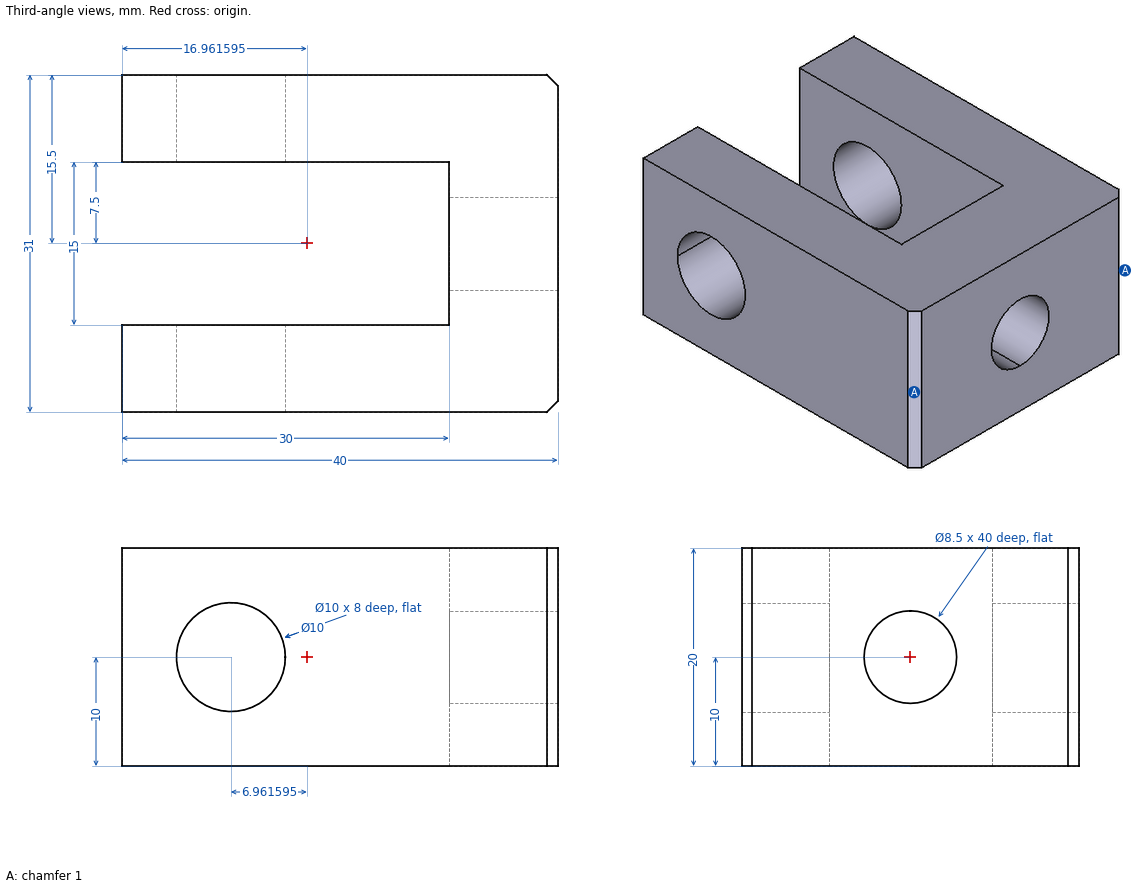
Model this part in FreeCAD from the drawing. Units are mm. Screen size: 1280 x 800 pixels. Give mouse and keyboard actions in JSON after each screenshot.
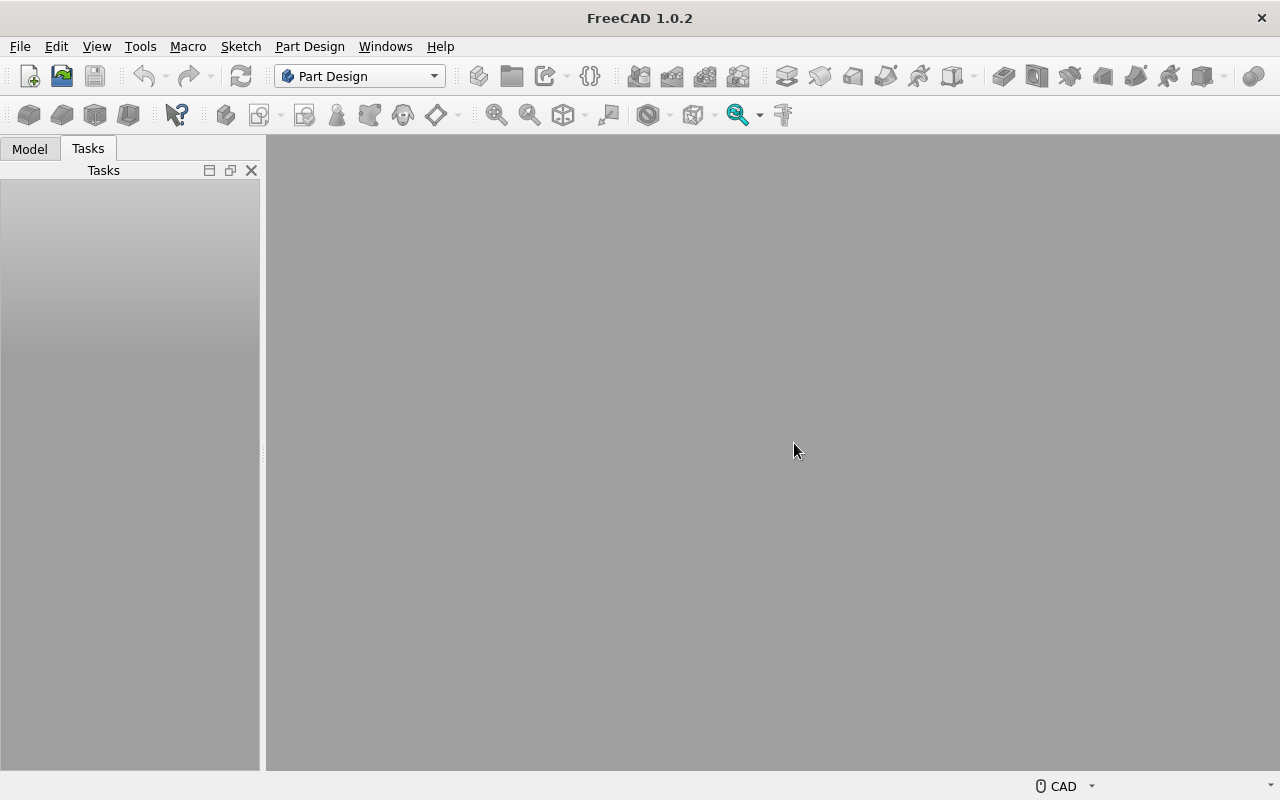
{"action": "left_click", "coordinate": [29, 76]}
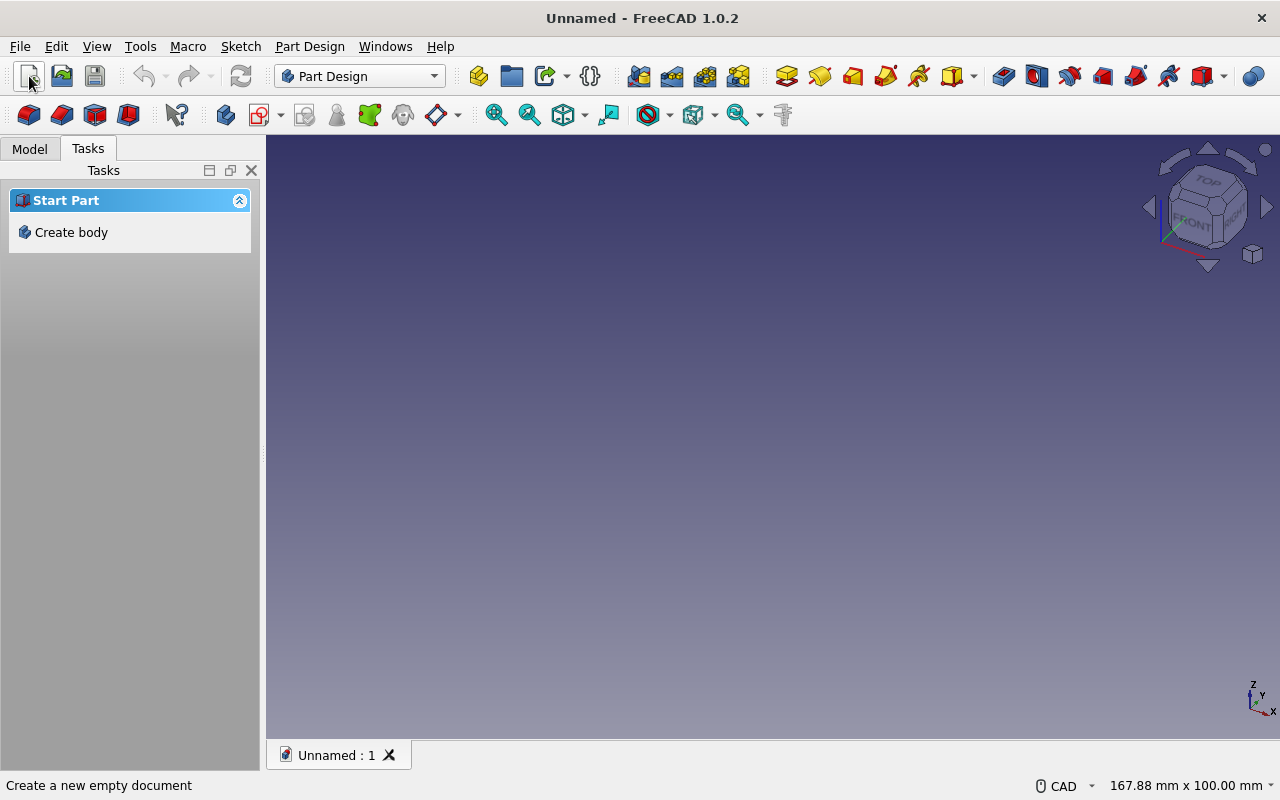
{"action": "left_click", "coordinate": [226, 116]}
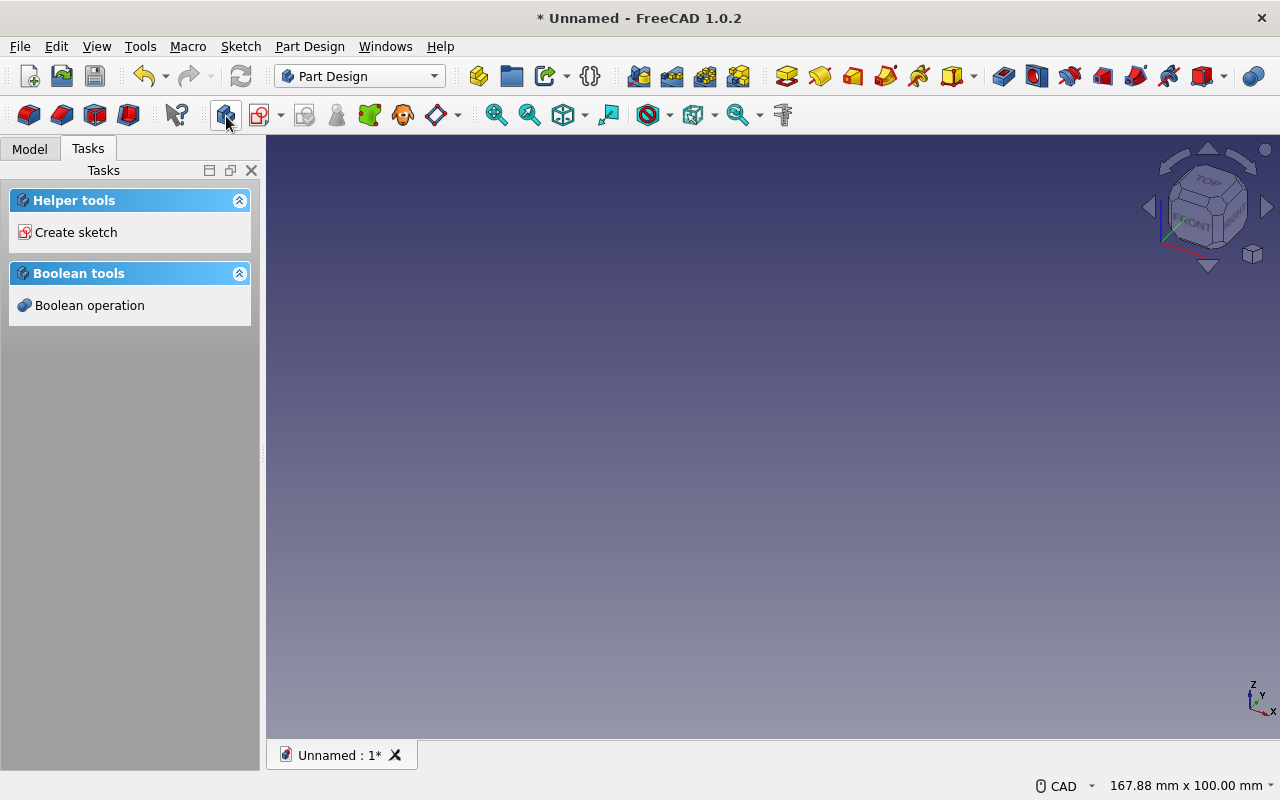
{"action": "left_click", "coordinate": [30, 148]}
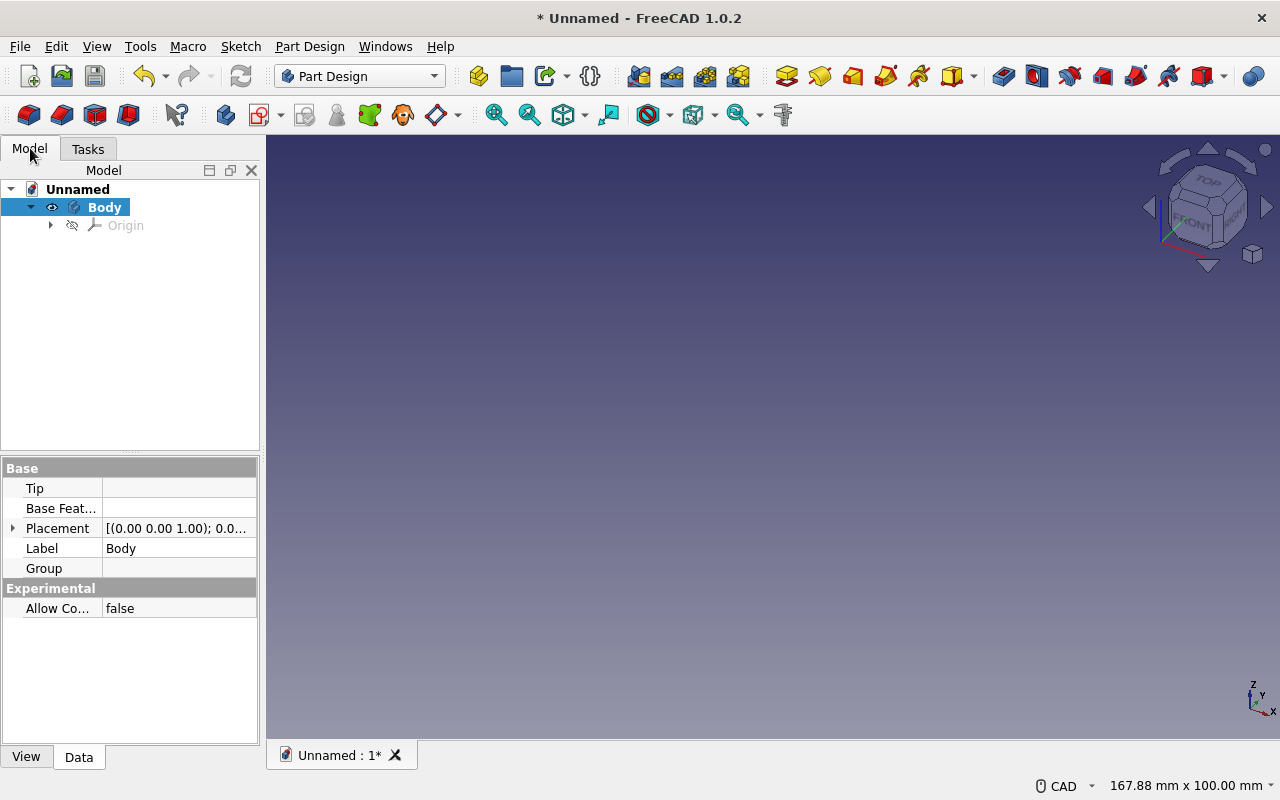
{"action": "left_click", "coordinate": [51, 225]}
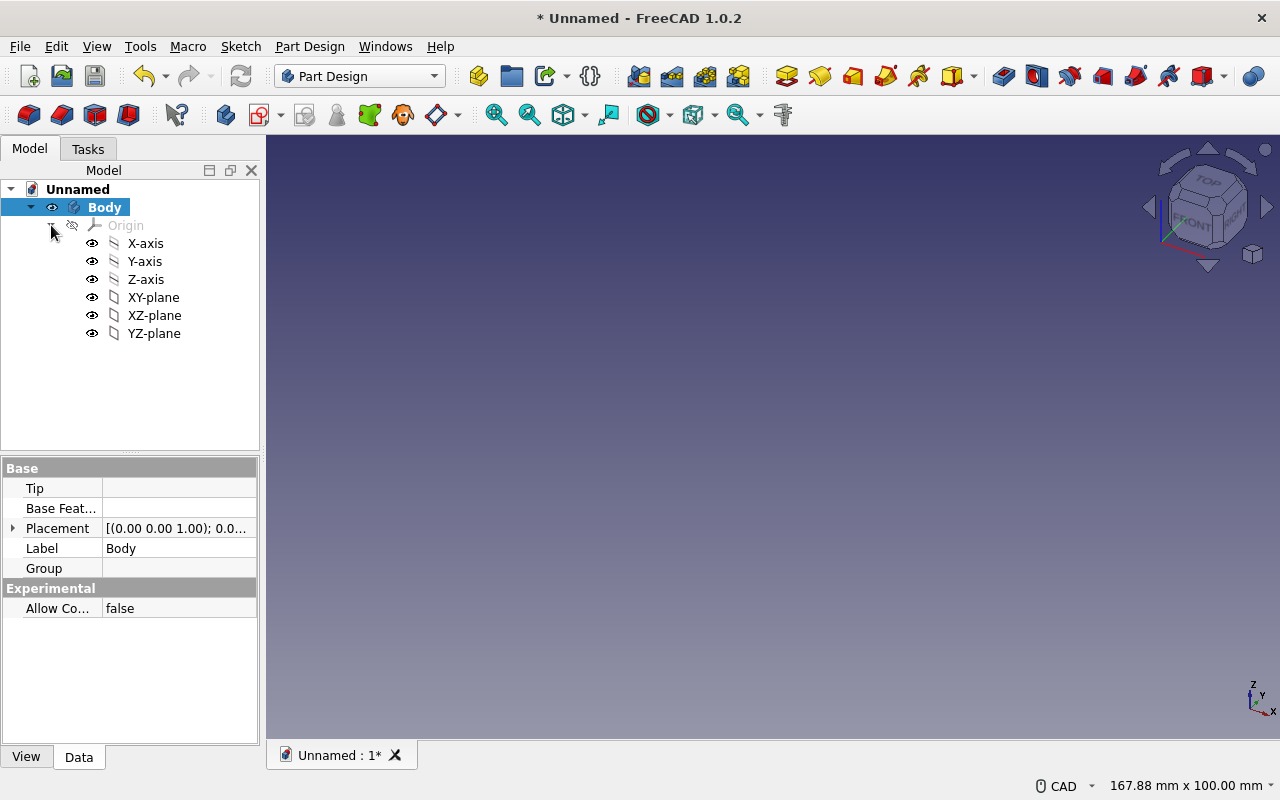
{"action": "left_click", "coordinate": [137, 297]}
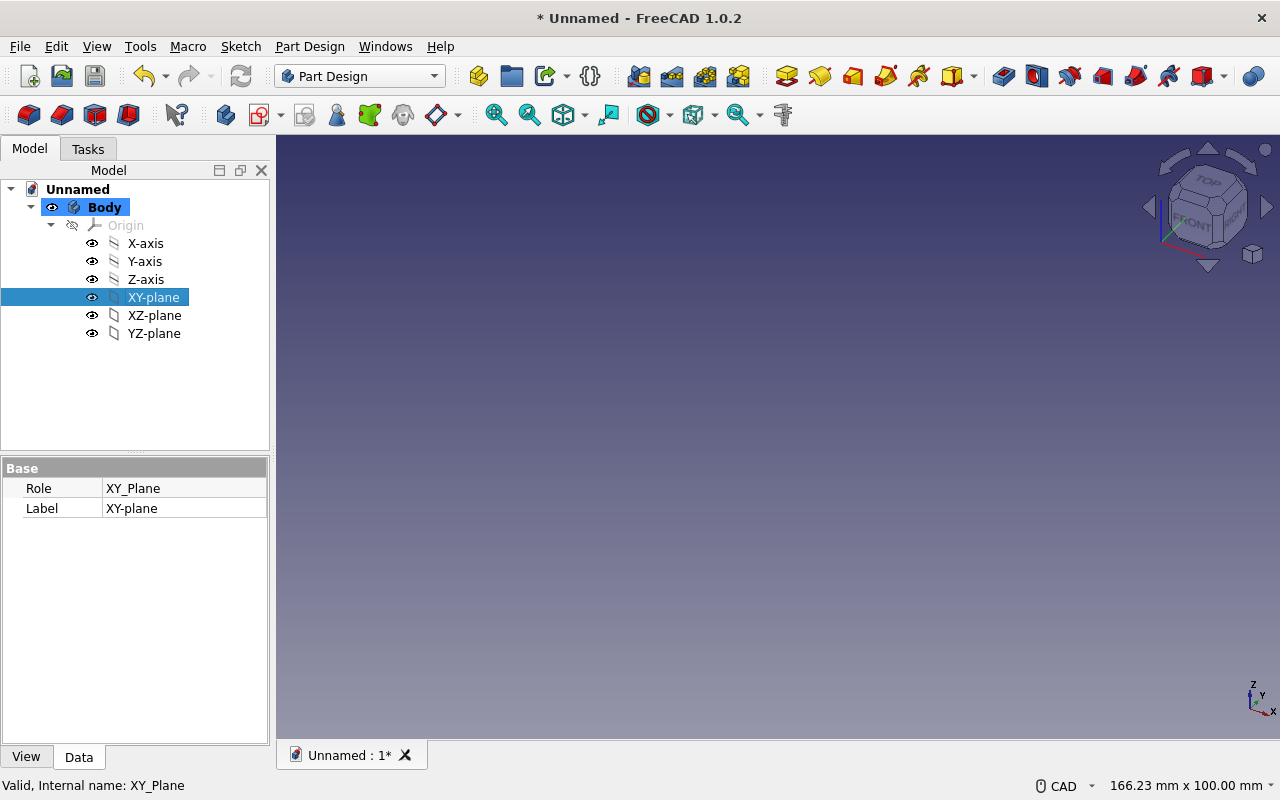
{"action": "left_click", "coordinate": [436, 116]}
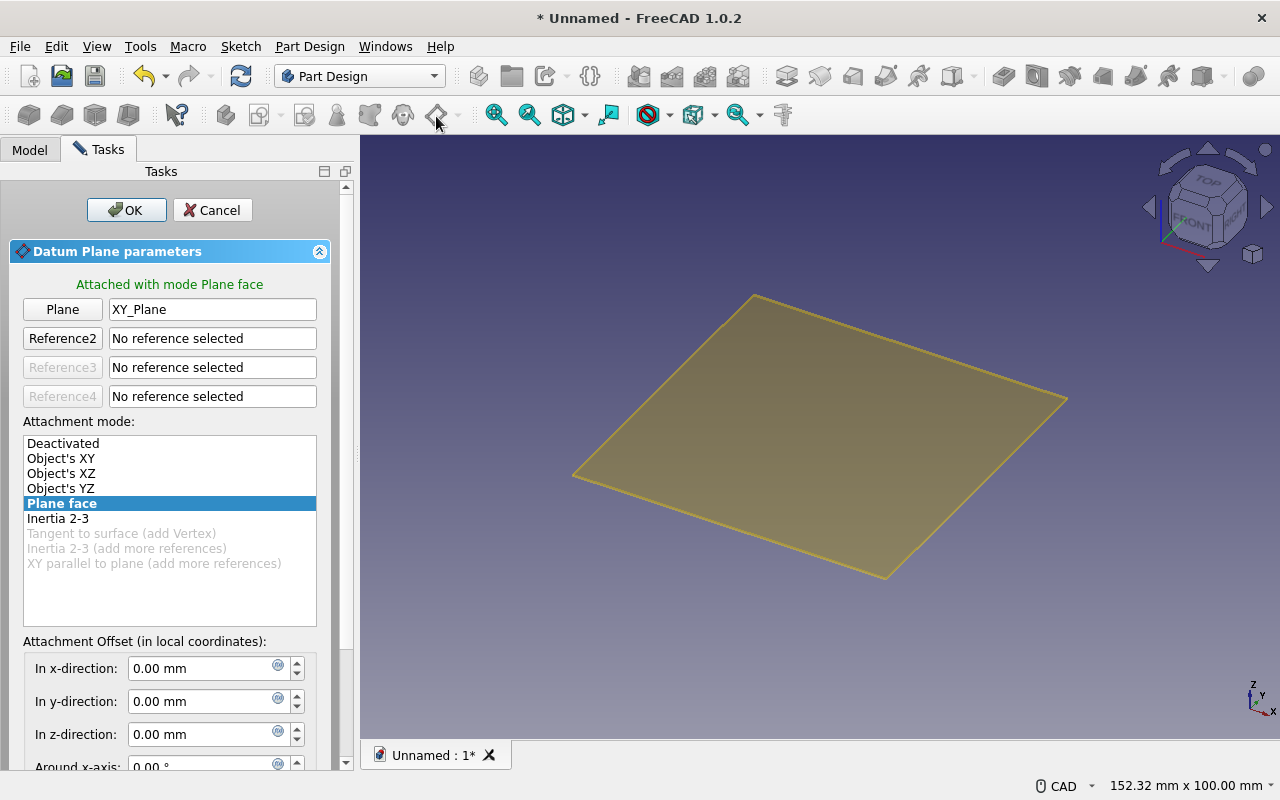
{"action": "triple_click", "coordinate": [210, 734]}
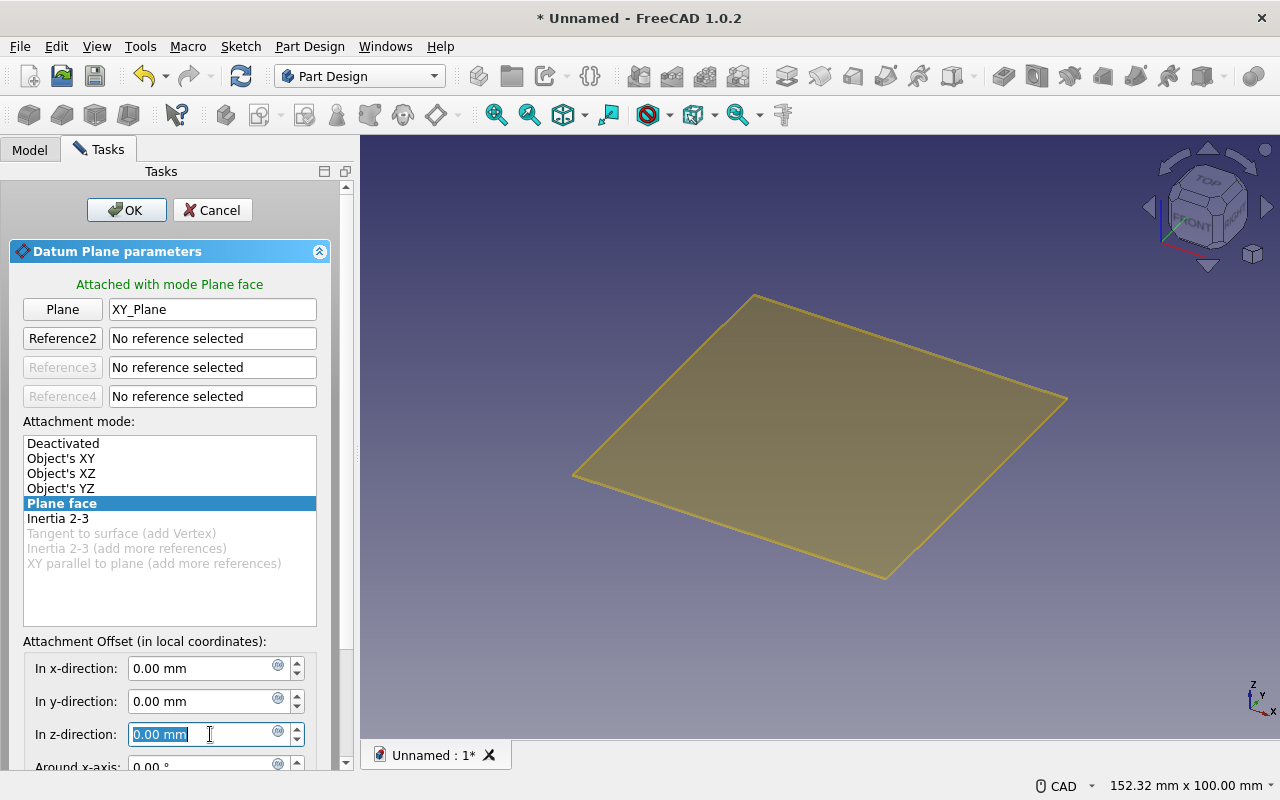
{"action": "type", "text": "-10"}
{"action": "key", "text": "Tab"}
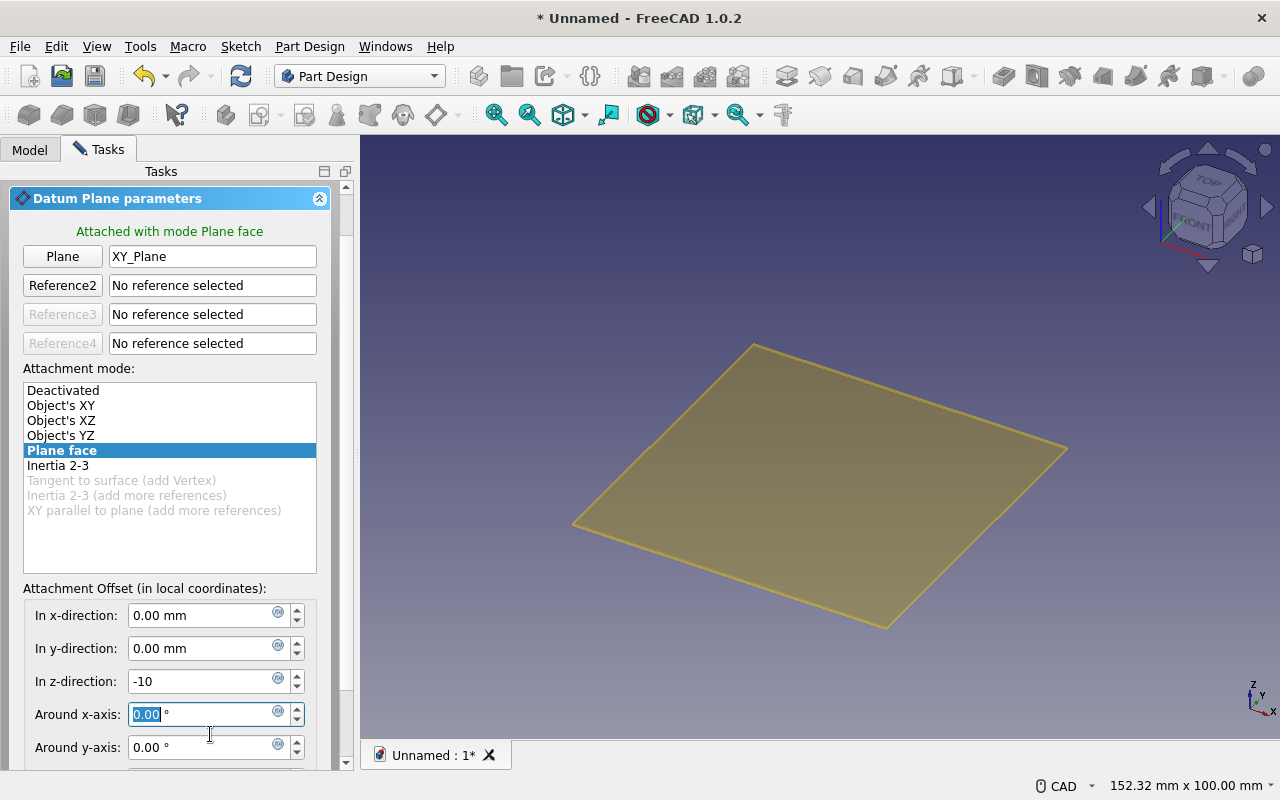
{"action": "scroll", "coordinate": [346, 476], "scroll_direction": "up", "scroll_amount": 2}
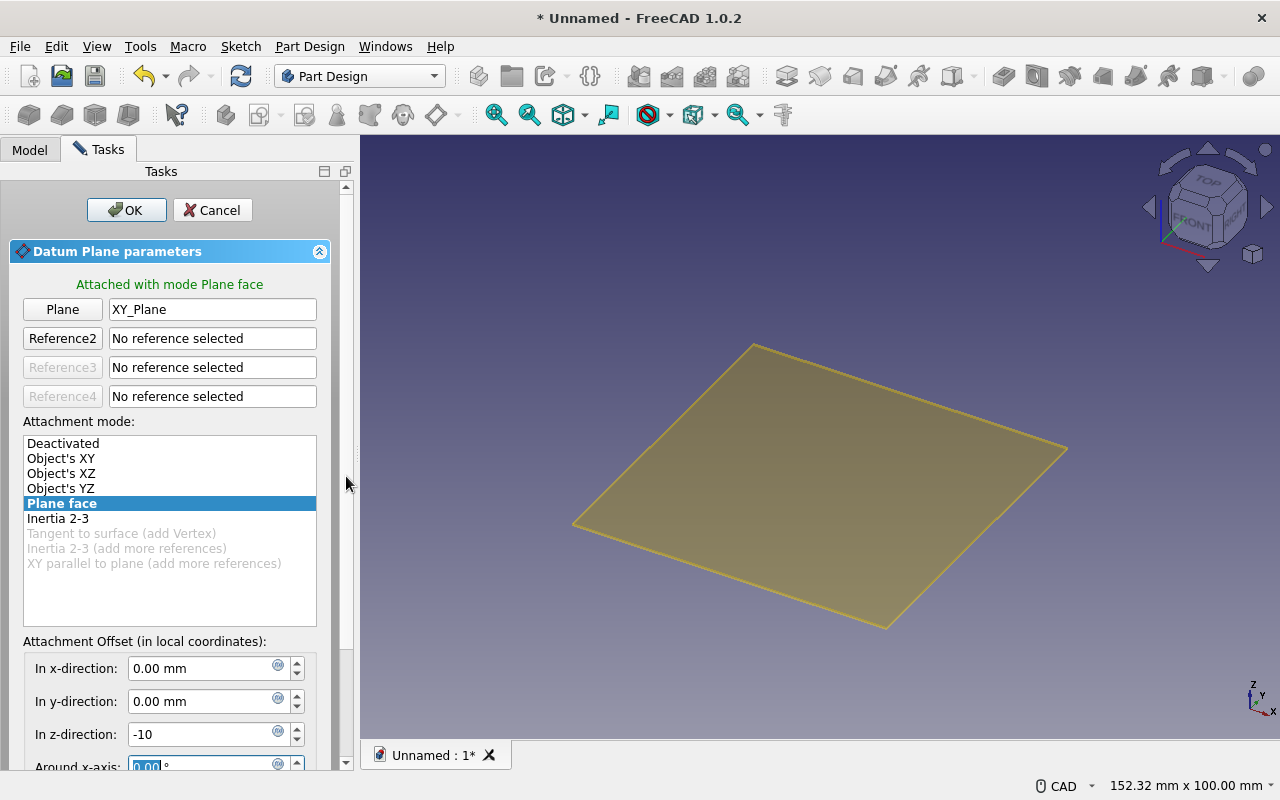
{"action": "left_click", "coordinate": [127, 210]}